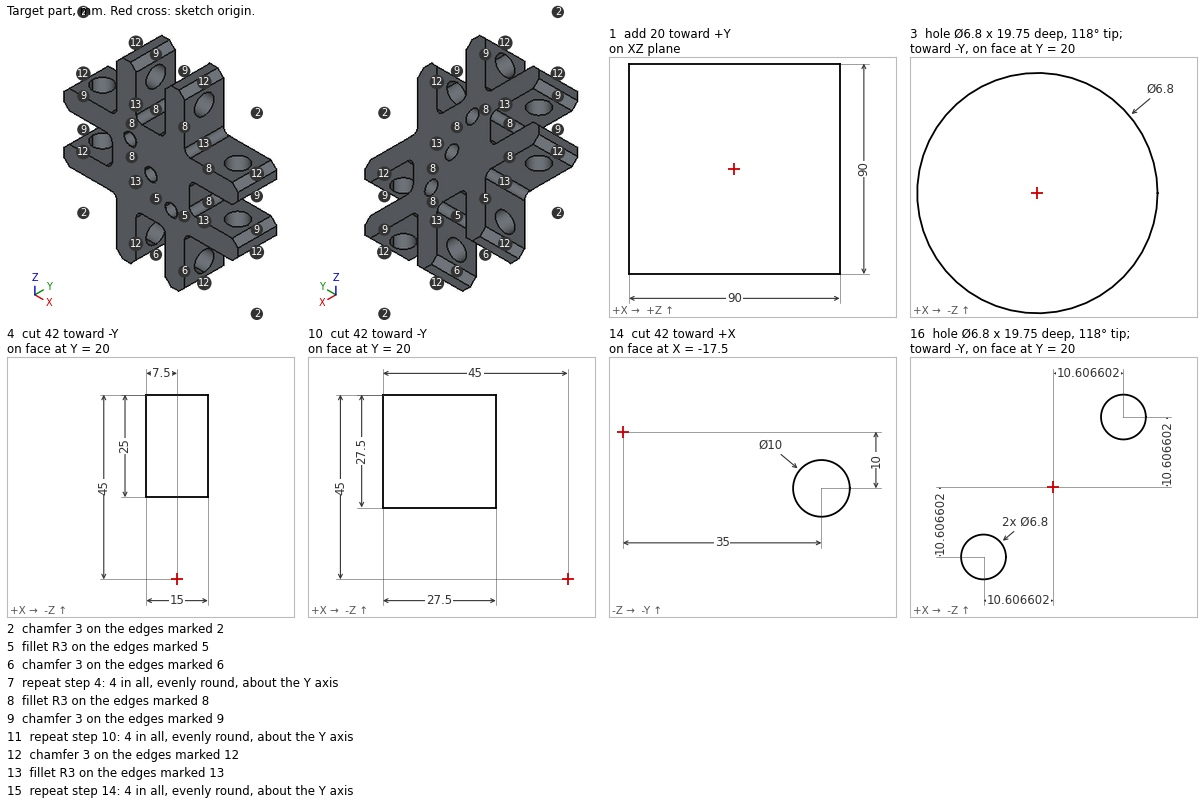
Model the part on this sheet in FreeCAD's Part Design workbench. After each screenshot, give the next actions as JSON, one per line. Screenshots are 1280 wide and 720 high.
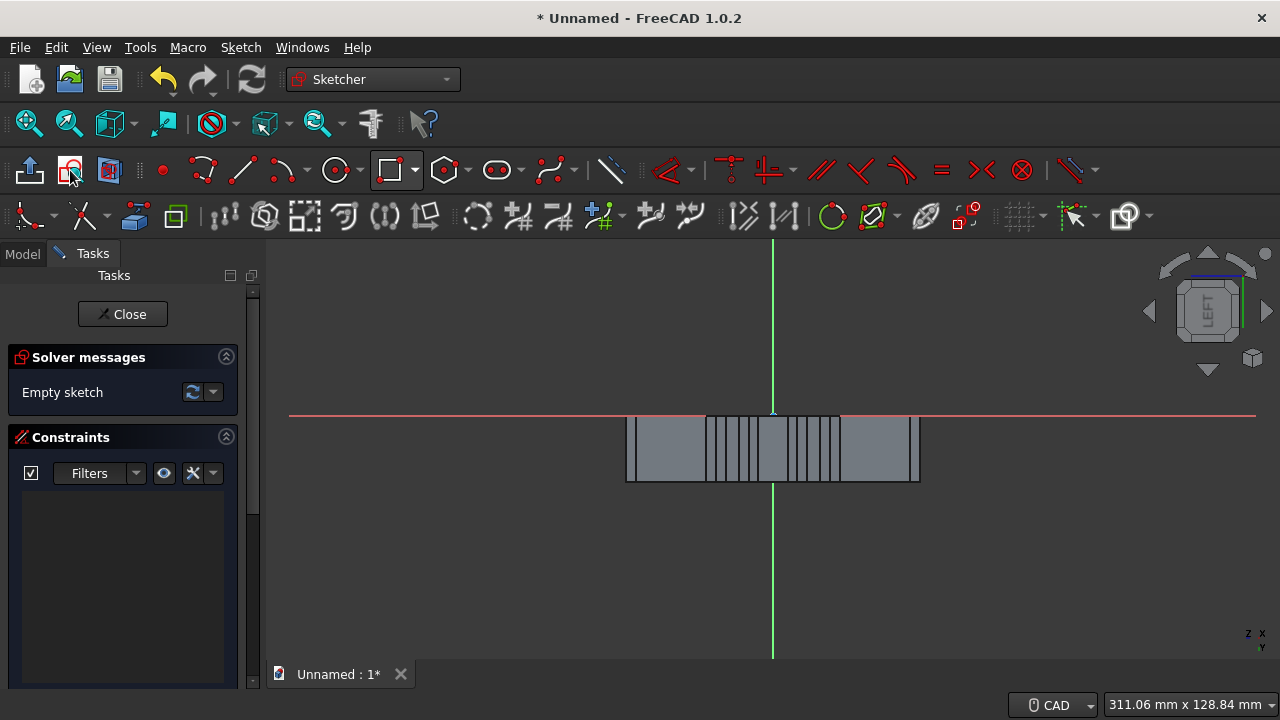
{"action": "scroll", "coordinate": [916, 449], "scroll_direction": "up", "scroll_amount": 10}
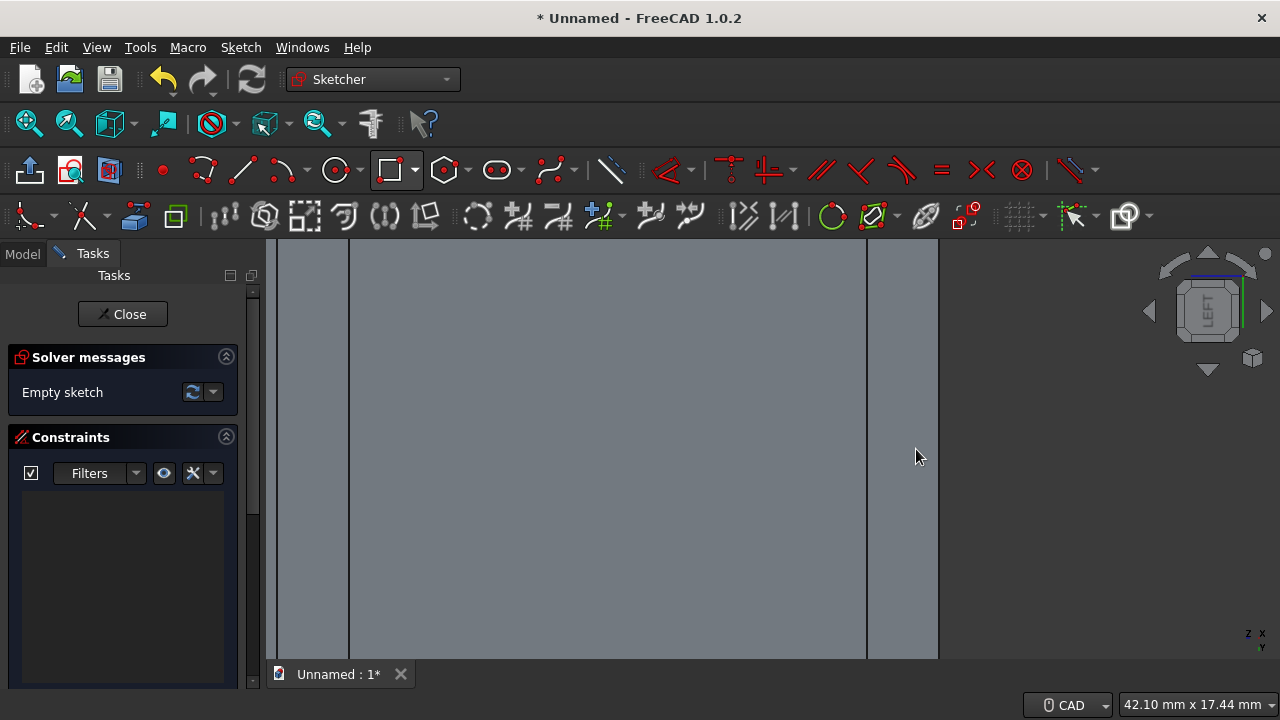
{"action": "left_click", "coordinate": [336, 170]}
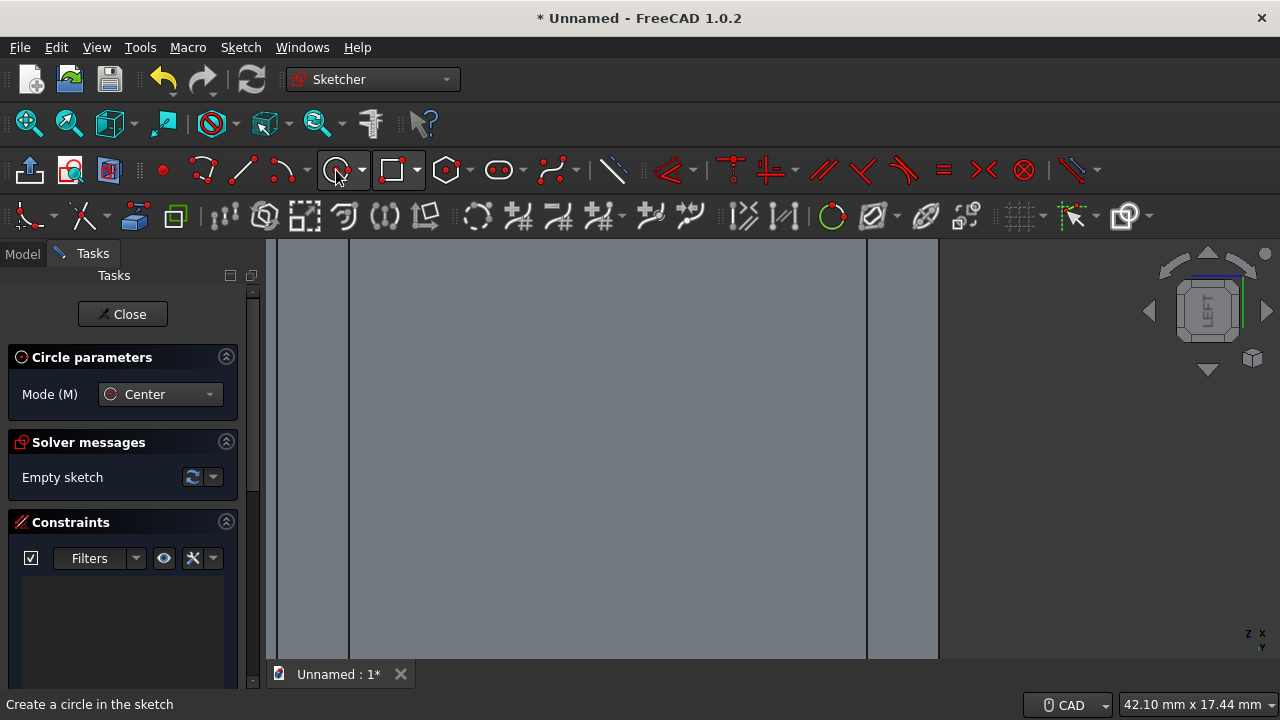
{"action": "left_click", "coordinate": [698, 446]}
{"action": "left_click", "coordinate": [783, 361]}
{"action": "key", "text": "Escape"}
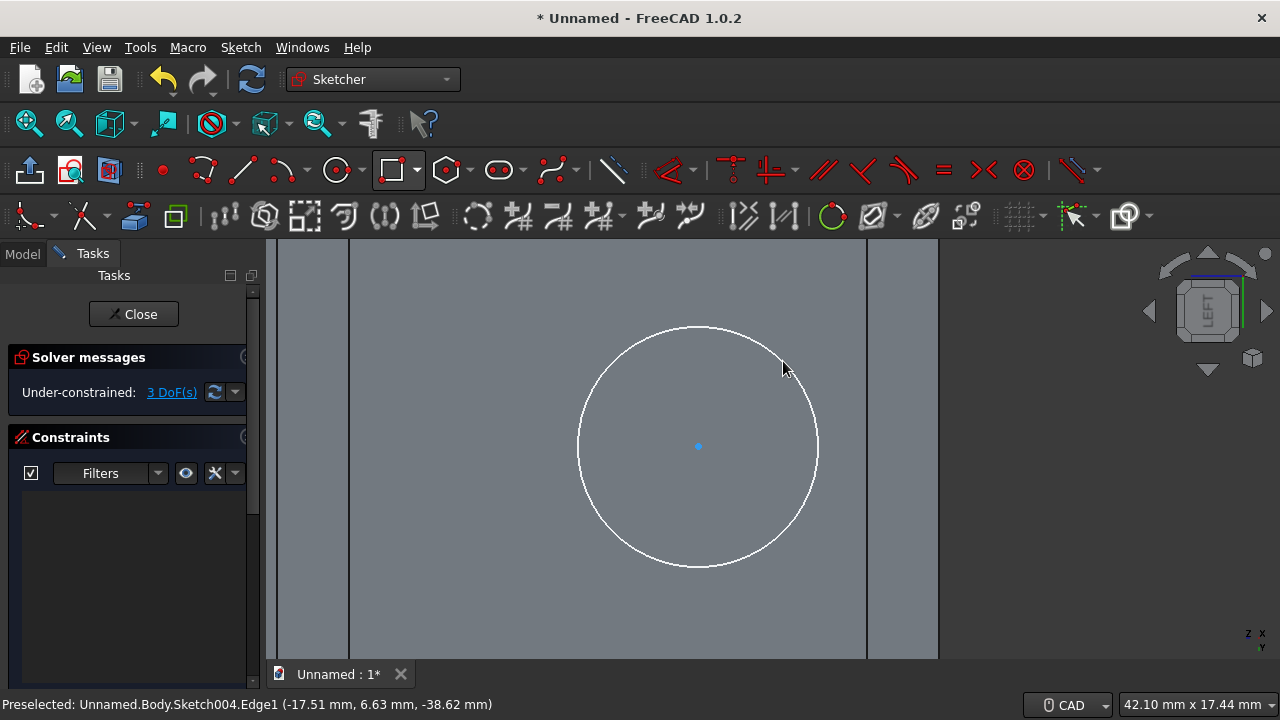
{"action": "left_click", "coordinate": [668, 170]}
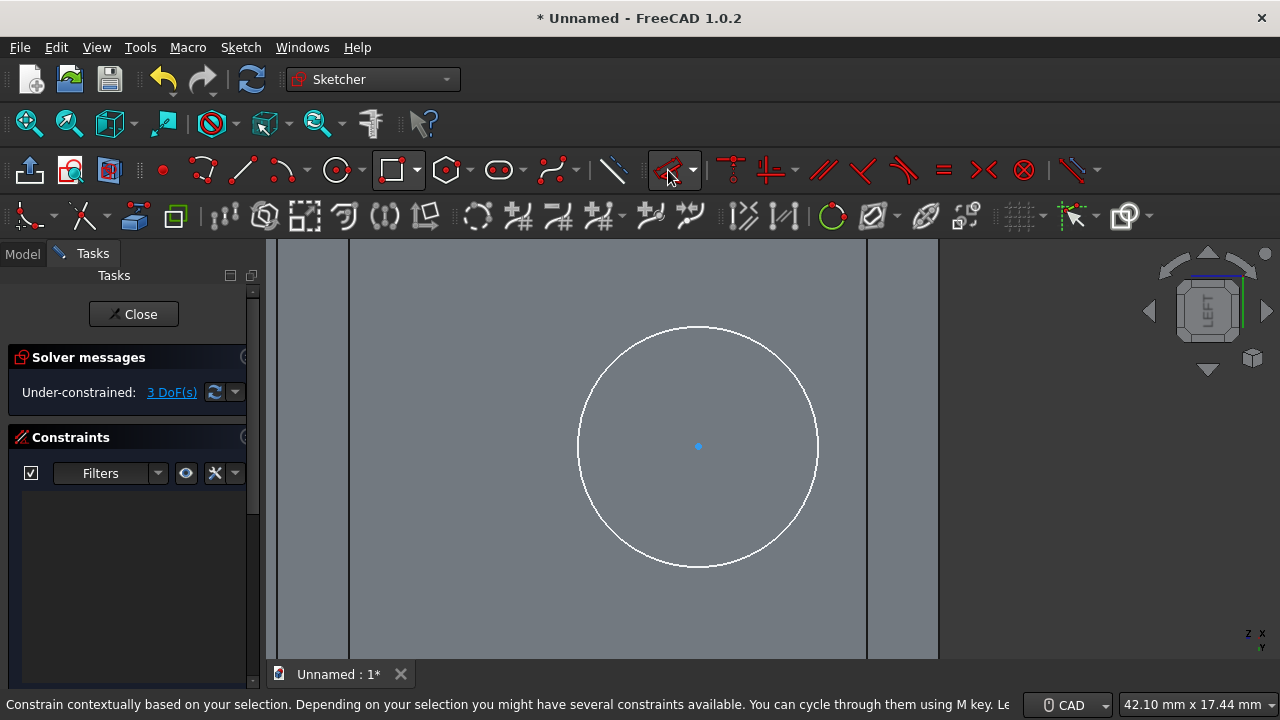
{"action": "left_click", "coordinate": [783, 362]}
{"action": "left_click", "coordinate": [806, 339]}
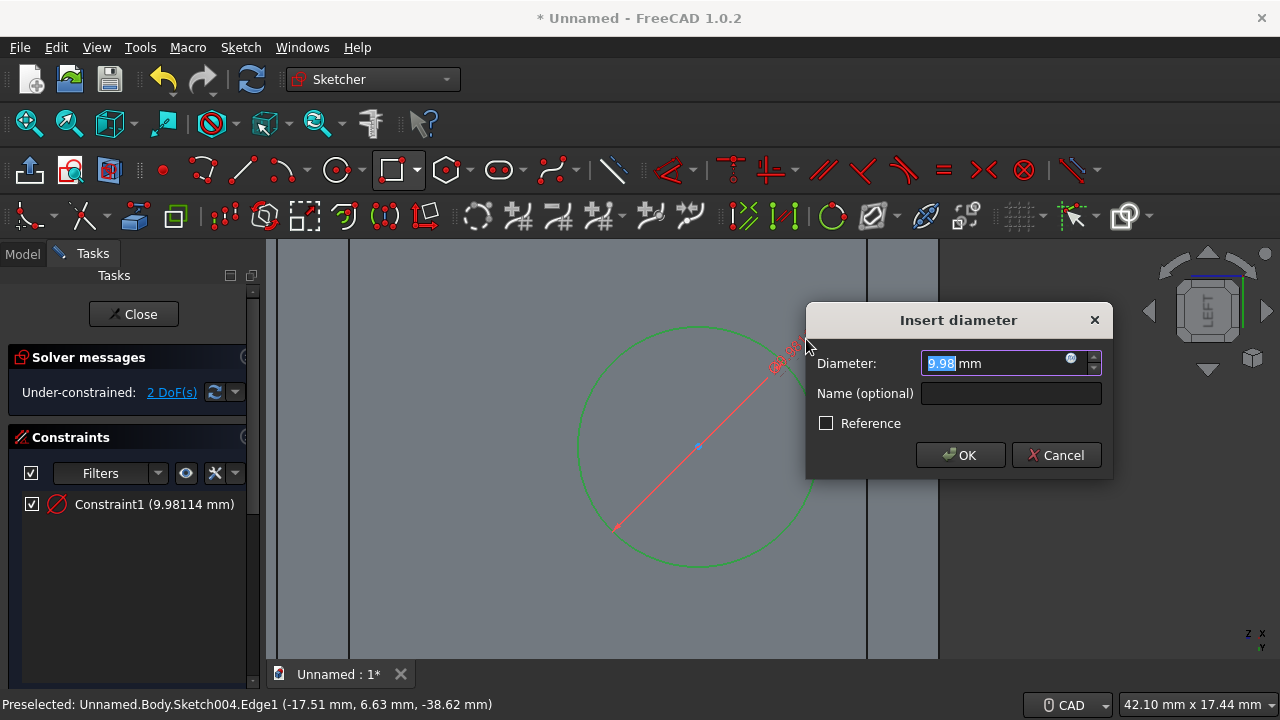
{"action": "type", "text": "10"}
{"action": "key", "text": "Return"}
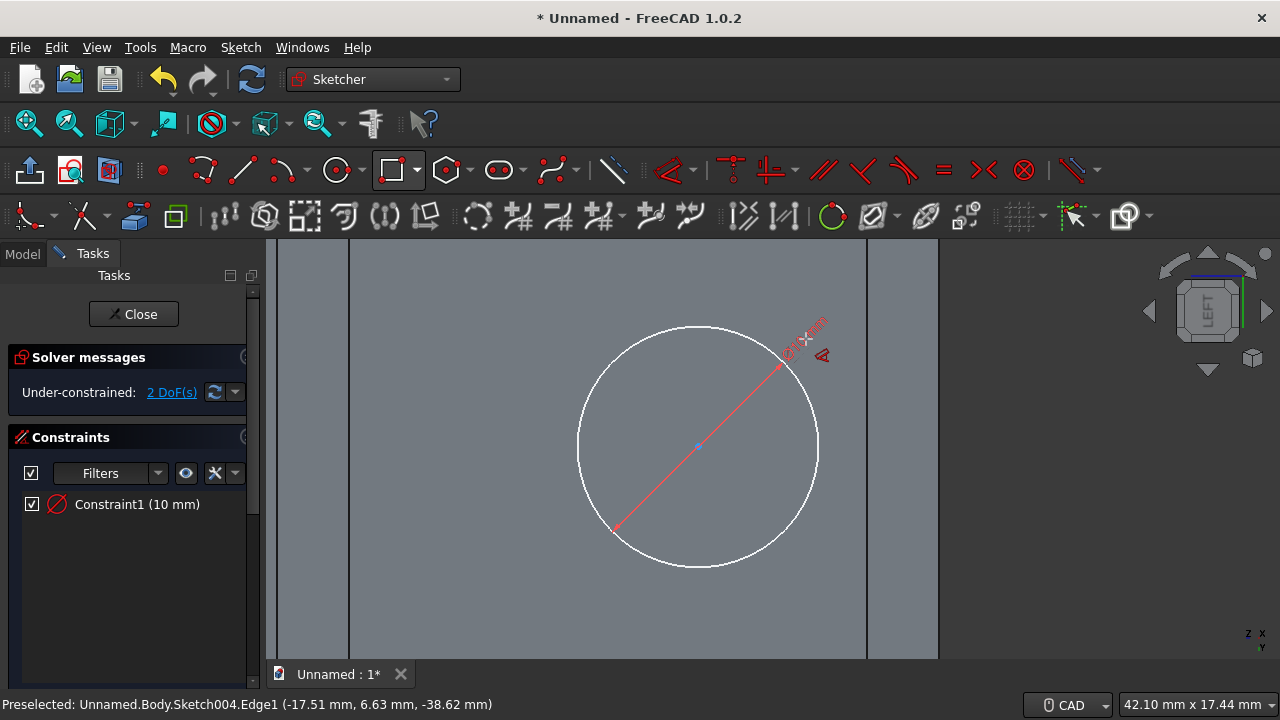
{"action": "left_click", "coordinate": [698, 447]}
{"action": "left_click", "coordinate": [496, 481]}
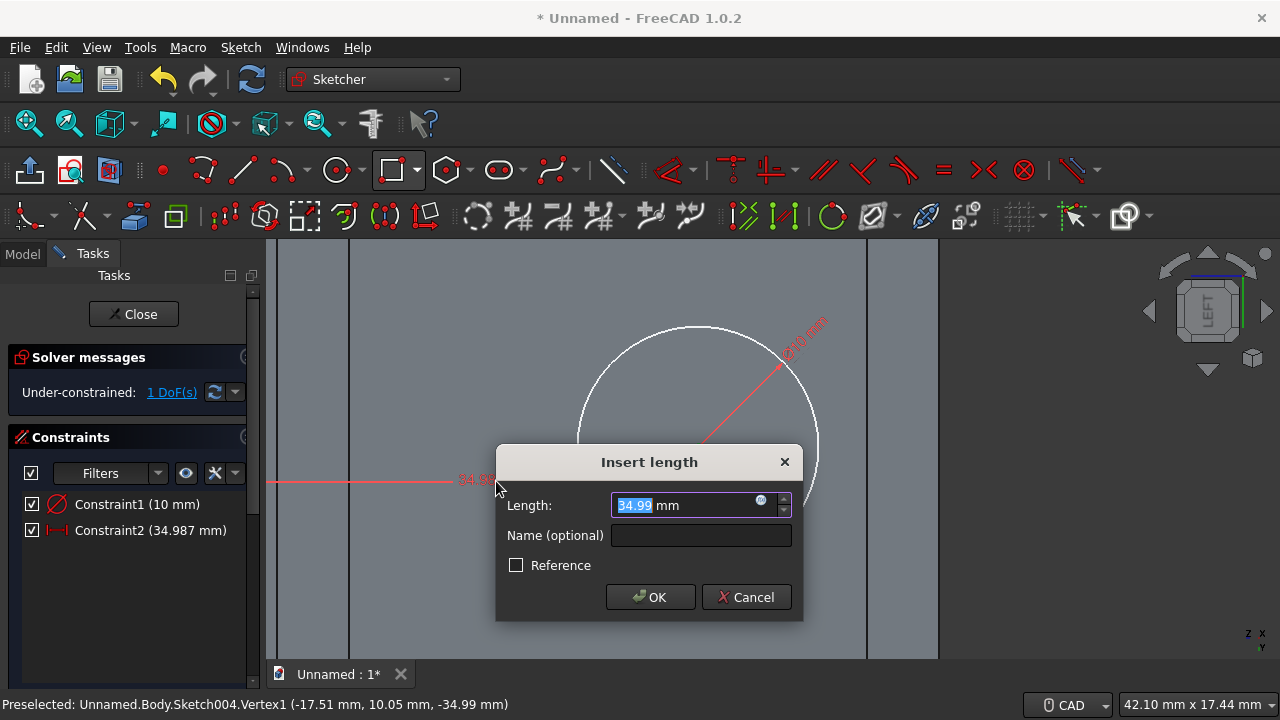
{"action": "type", "text": "35"}
{"action": "key", "text": "Return"}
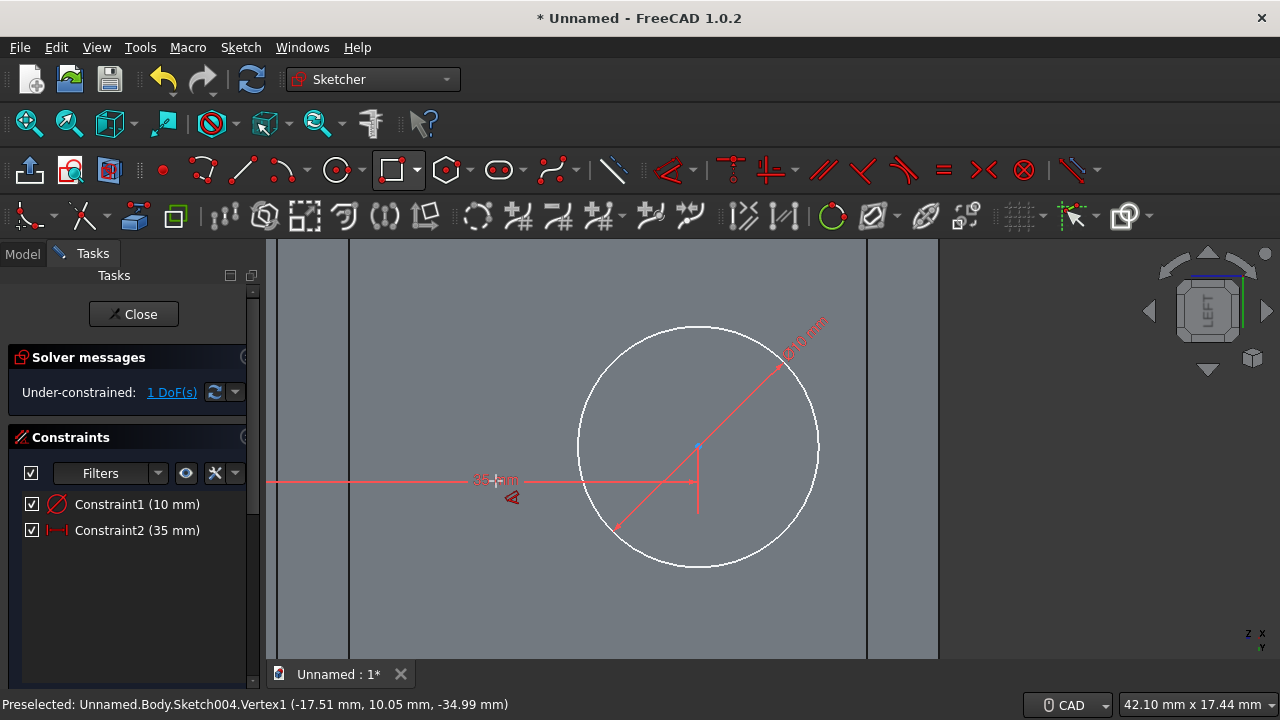
{"action": "left_click", "coordinate": [698, 447]}
{"action": "left_click", "coordinate": [732, 357]}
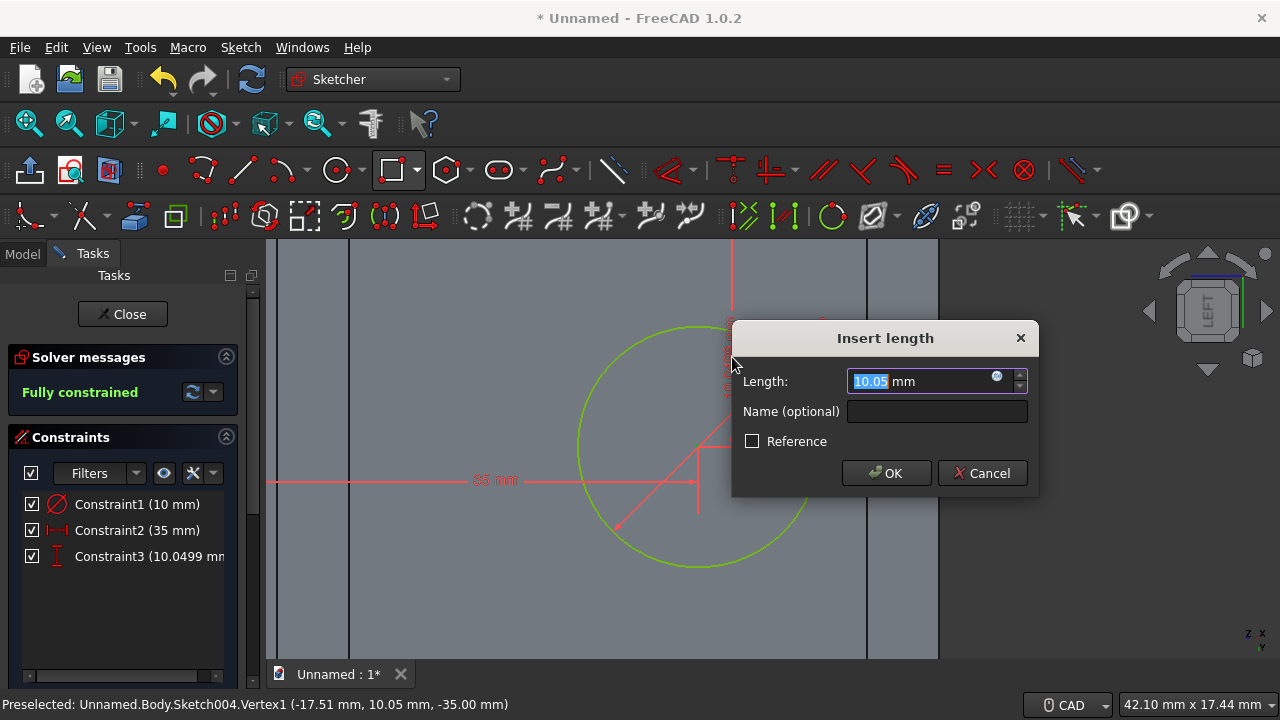
{"action": "type", "text": "10"}
{"action": "key", "text": "Return"}
{"action": "key", "text": "Escape"}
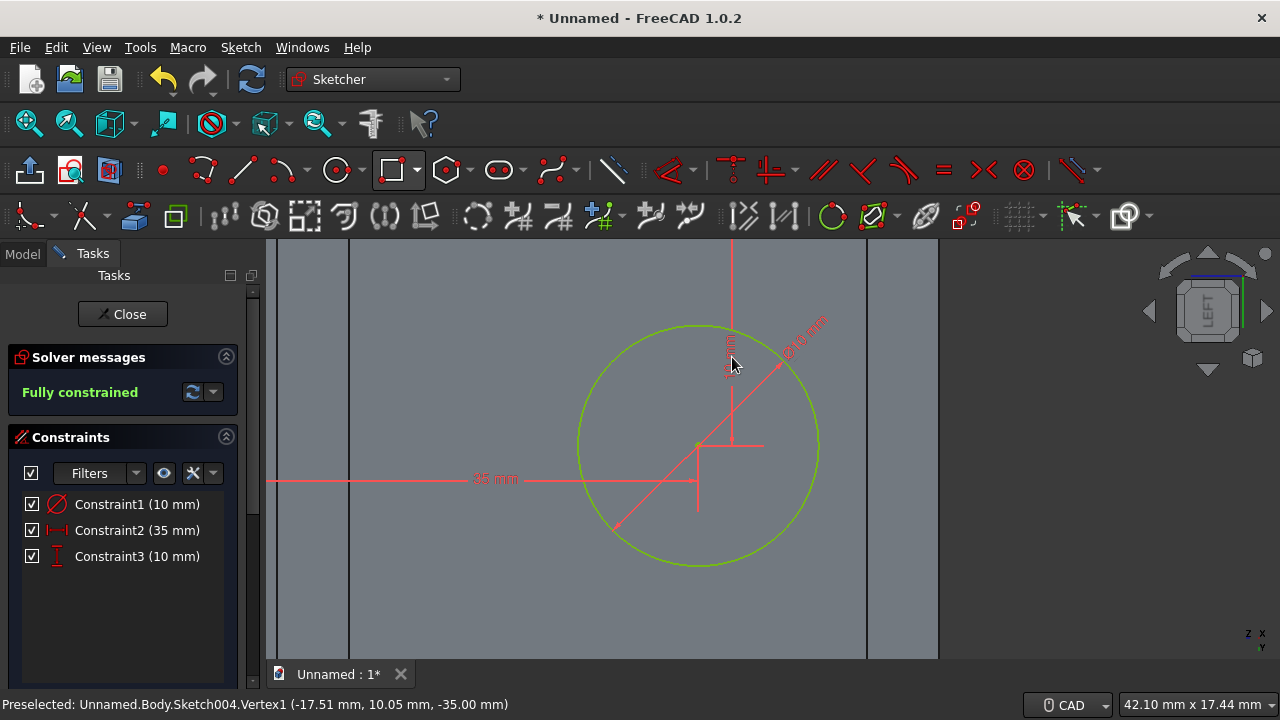
{"action": "left_click", "coordinate": [123, 314]}